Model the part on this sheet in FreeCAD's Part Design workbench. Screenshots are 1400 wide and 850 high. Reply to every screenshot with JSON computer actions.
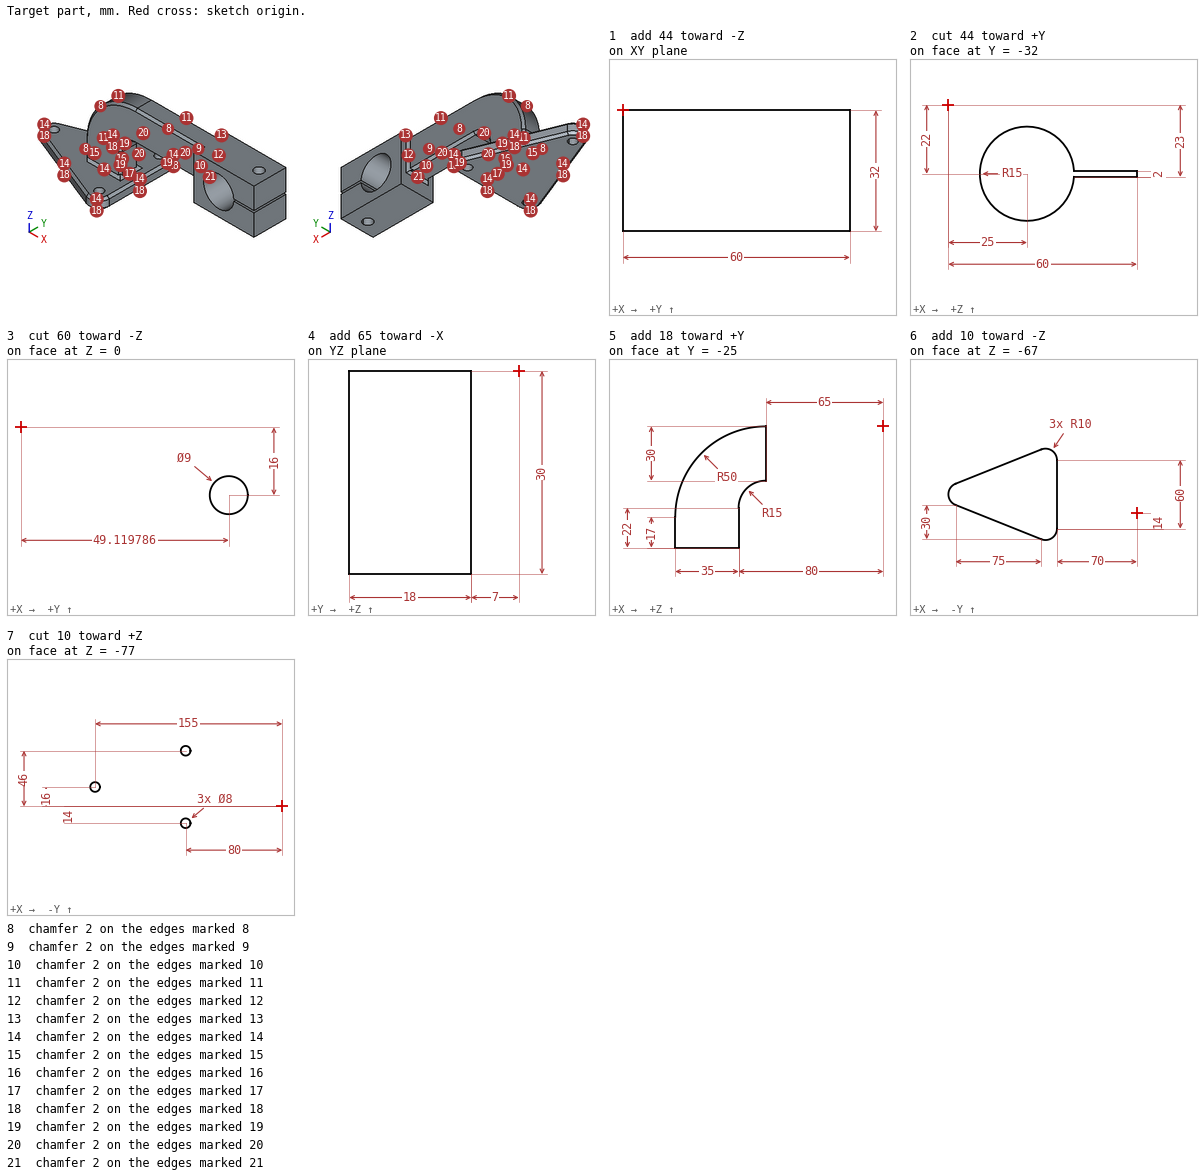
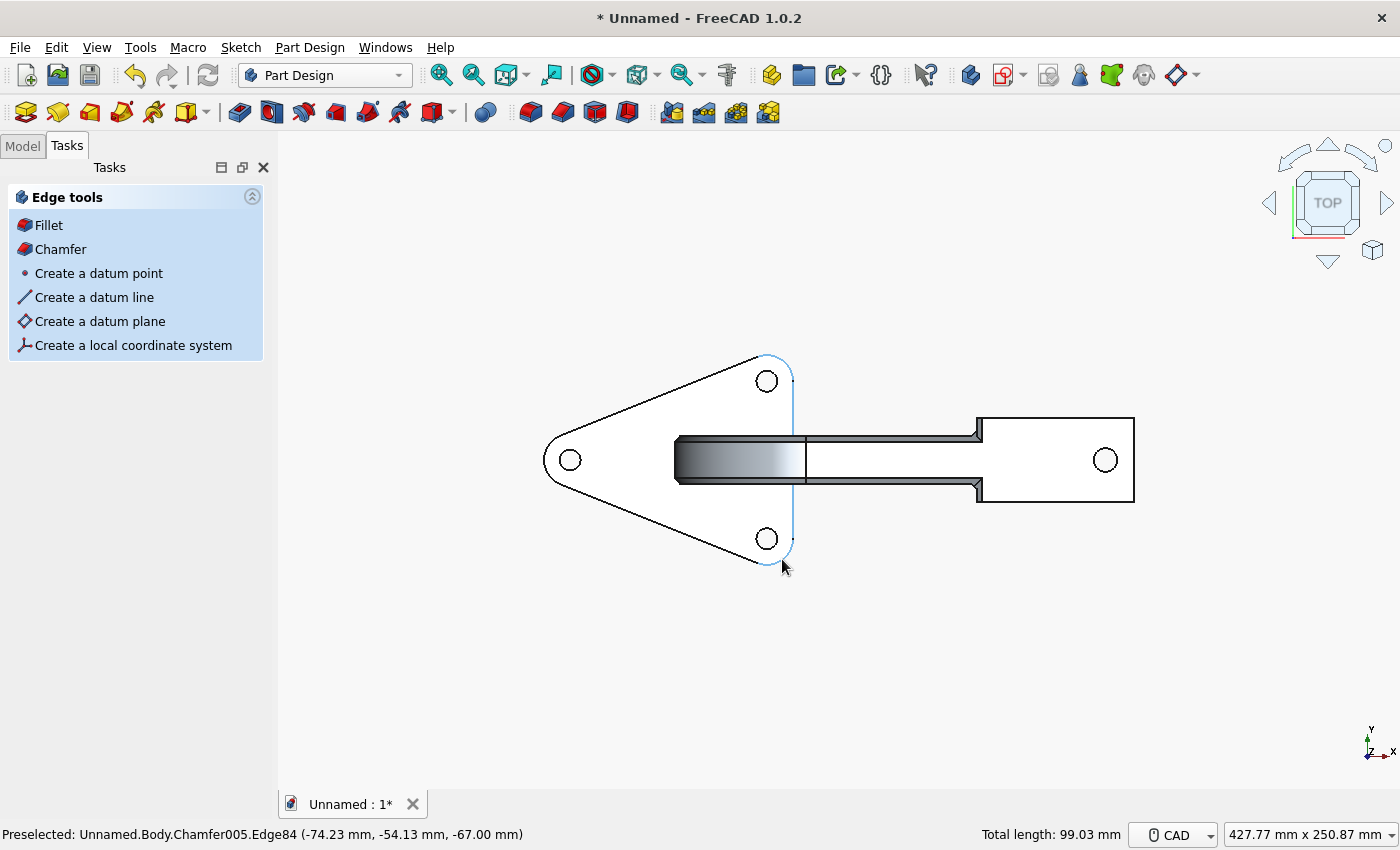
{"action": "left_click", "coordinate": [659, 523], "text": "ctrl"}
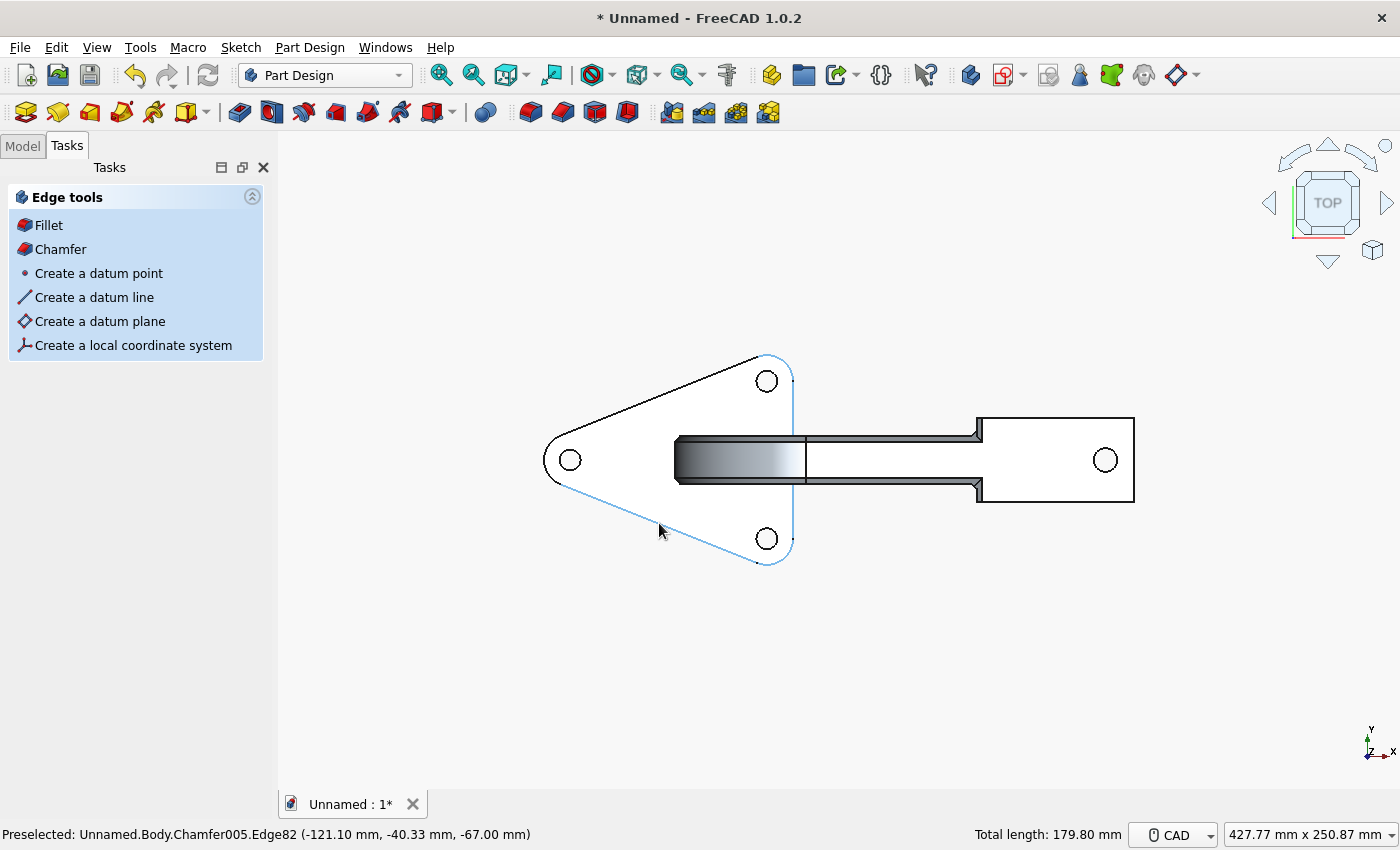
{"action": "left_click", "coordinate": [544, 459], "text": "ctrl"}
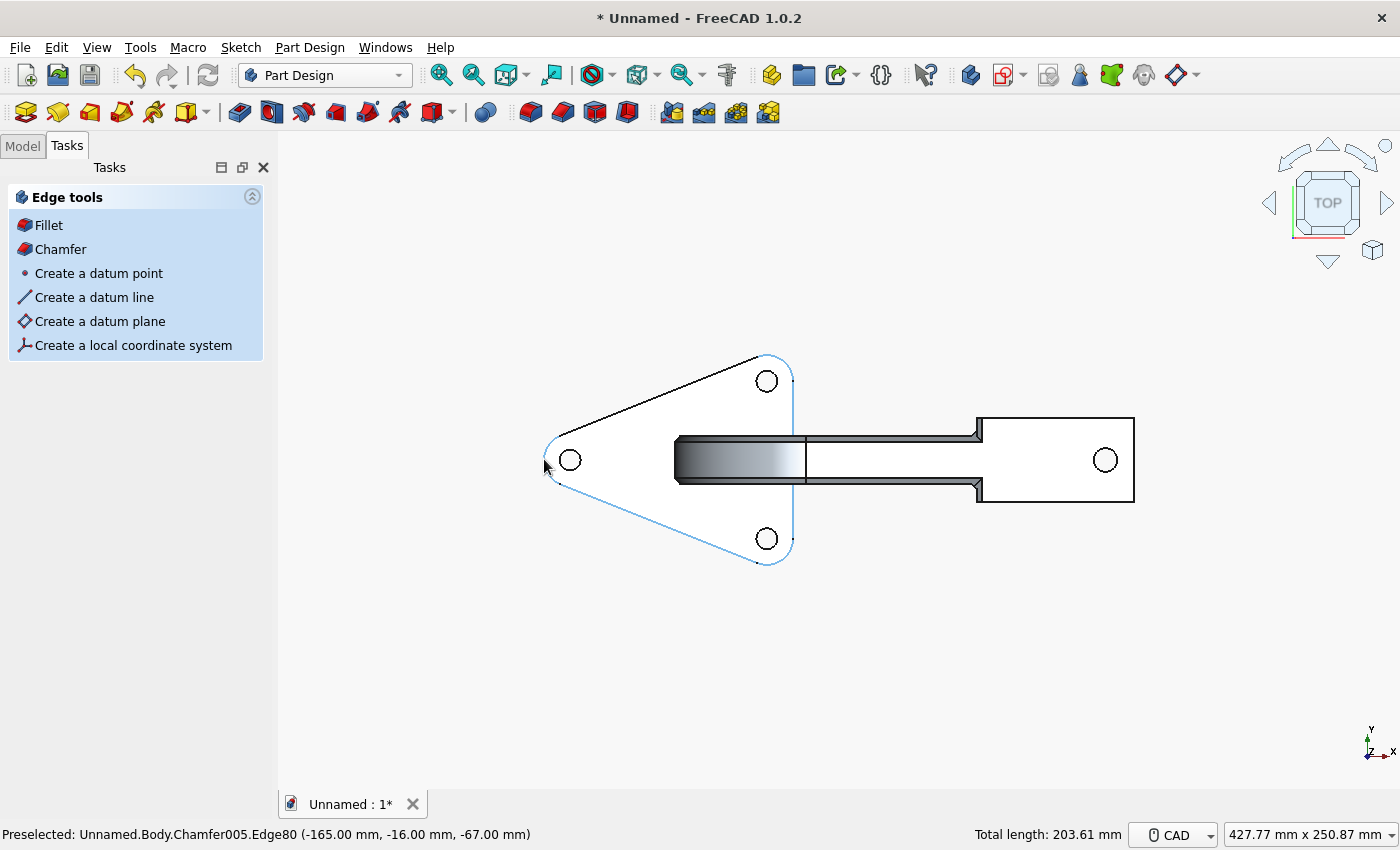
{"action": "left_click", "coordinate": [659, 395], "text": "ctrl"}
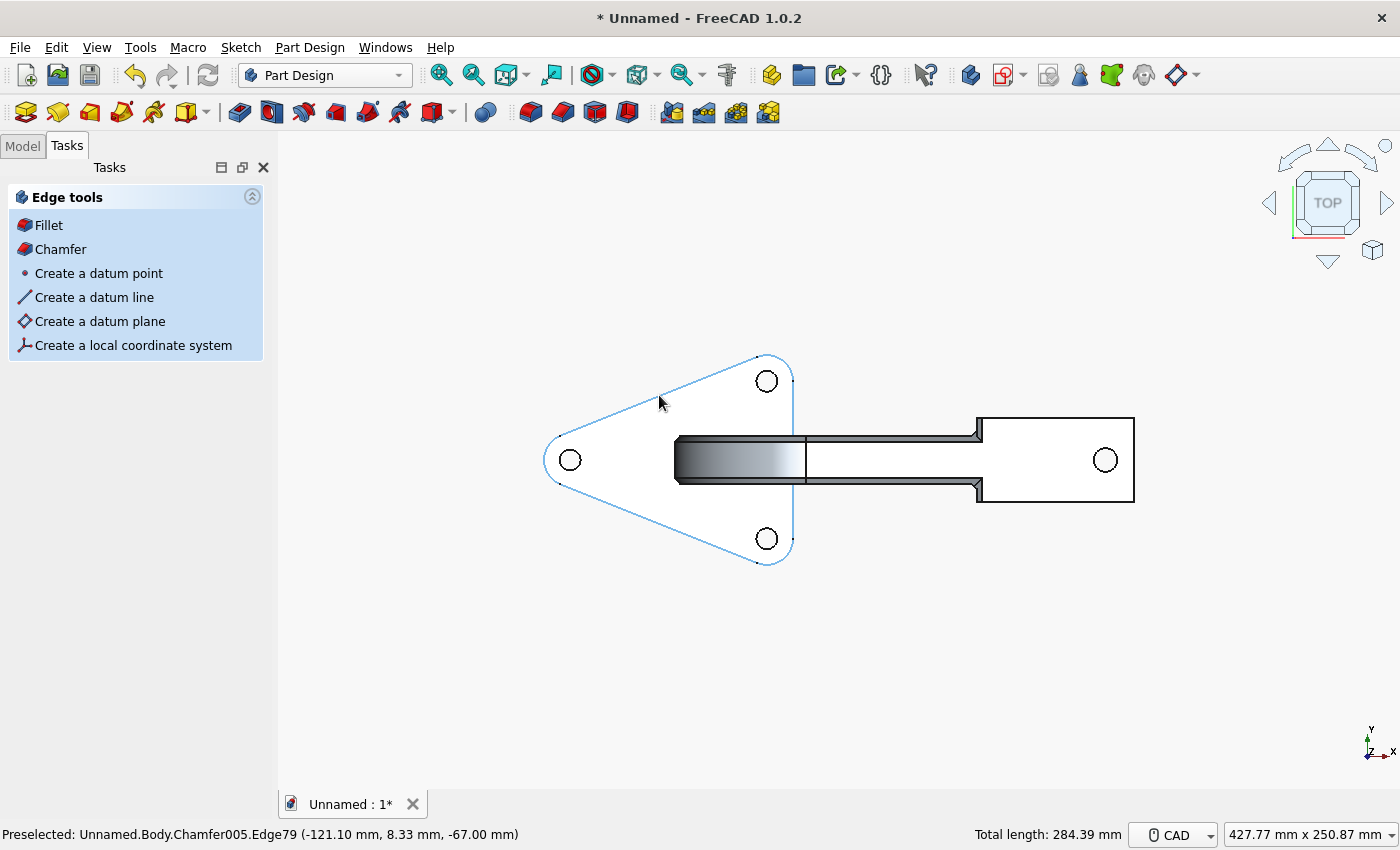
{"action": "key", "text": "0"}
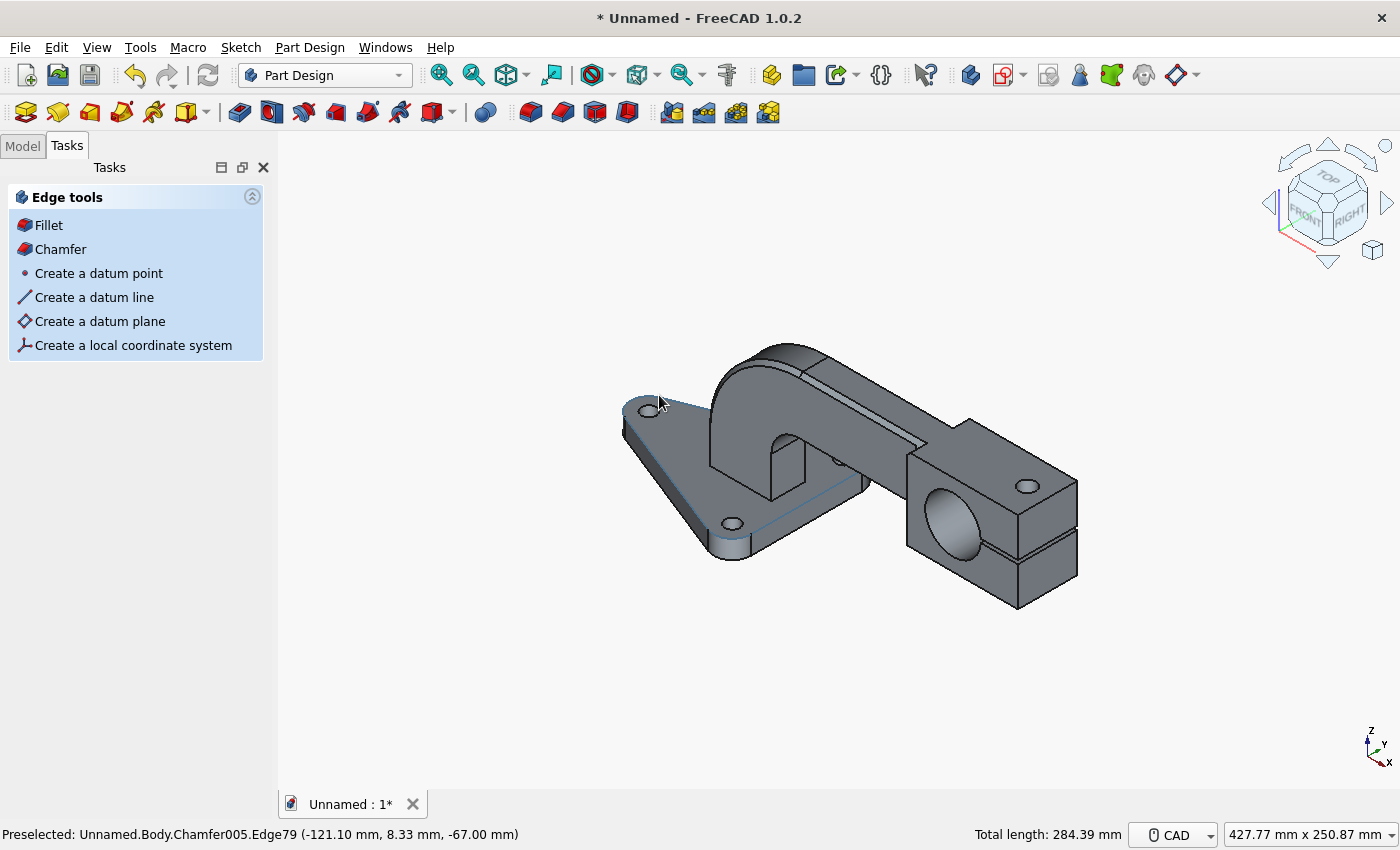
{"action": "key", "text": "2"}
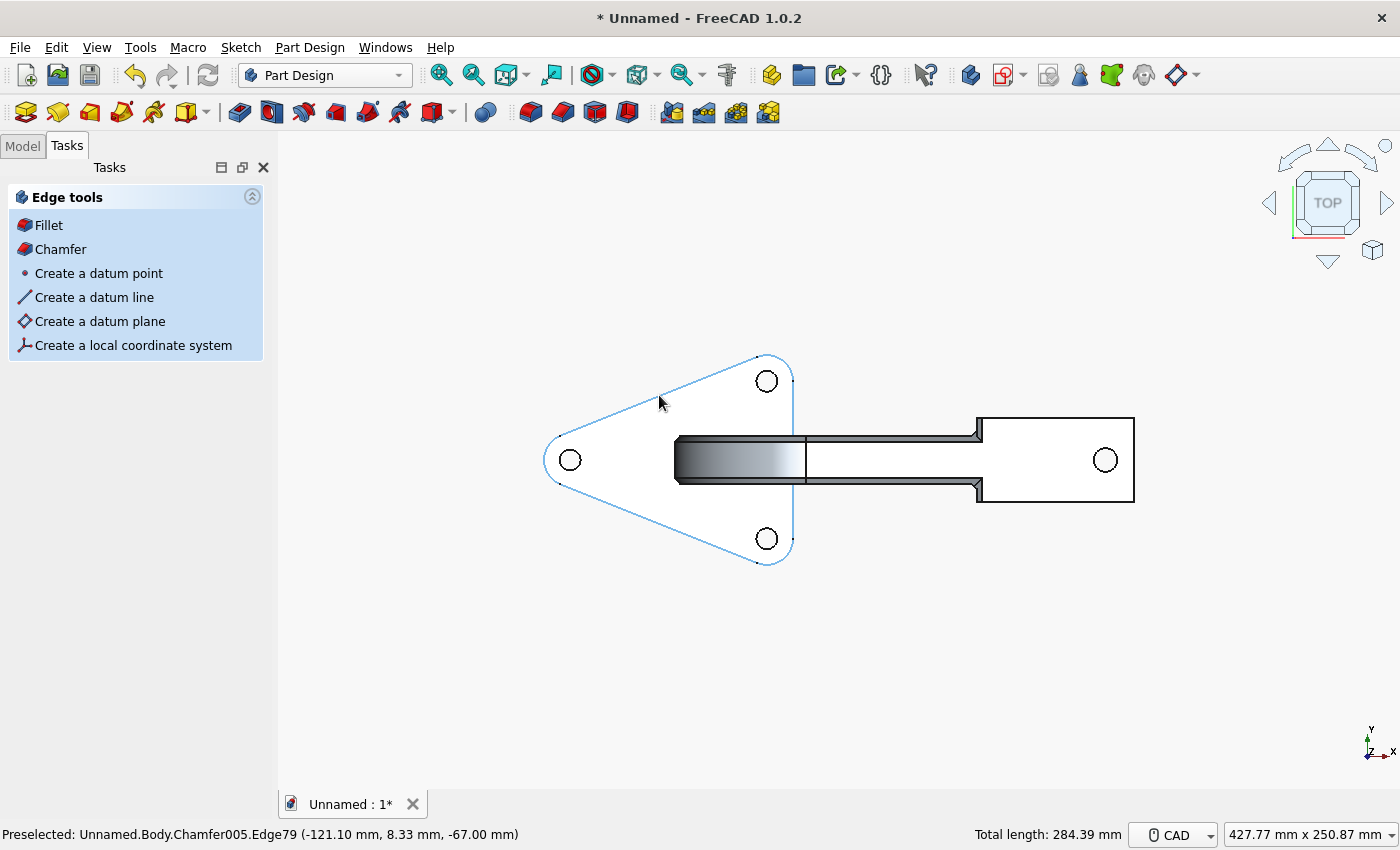
{"action": "key", "text": "1"}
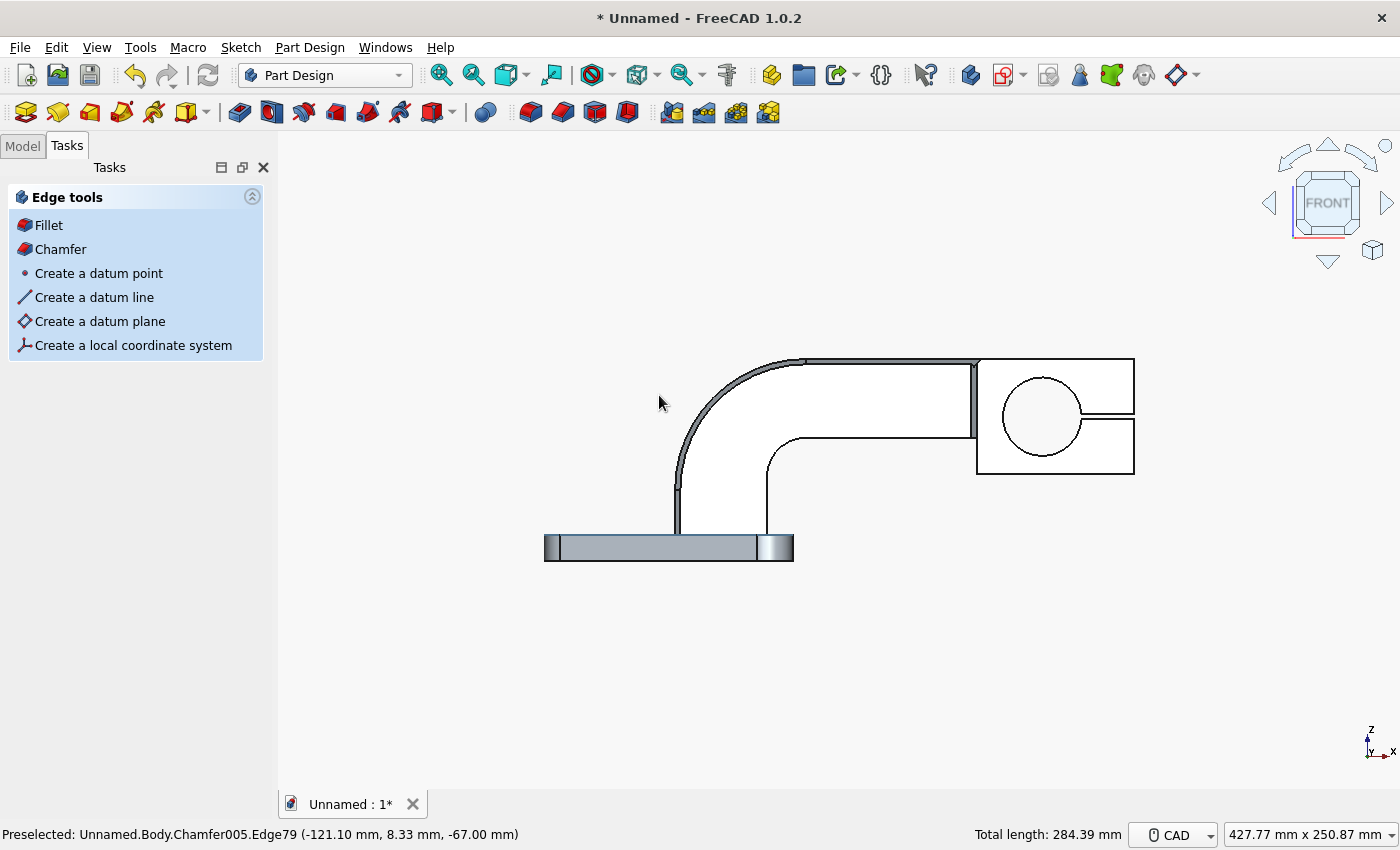
{"action": "key", "text": "3"}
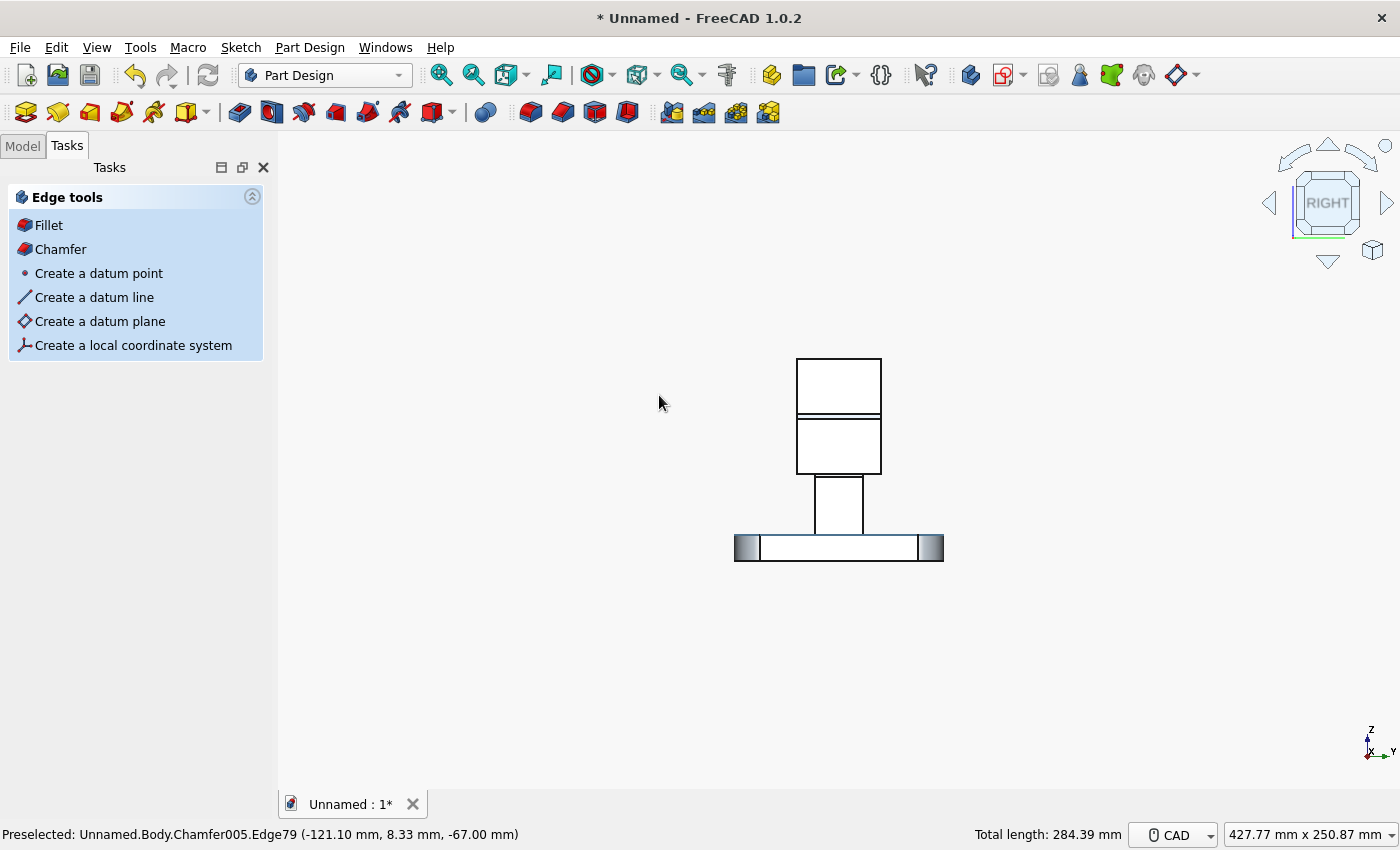
{"action": "left_click", "coordinate": [442, 76]}